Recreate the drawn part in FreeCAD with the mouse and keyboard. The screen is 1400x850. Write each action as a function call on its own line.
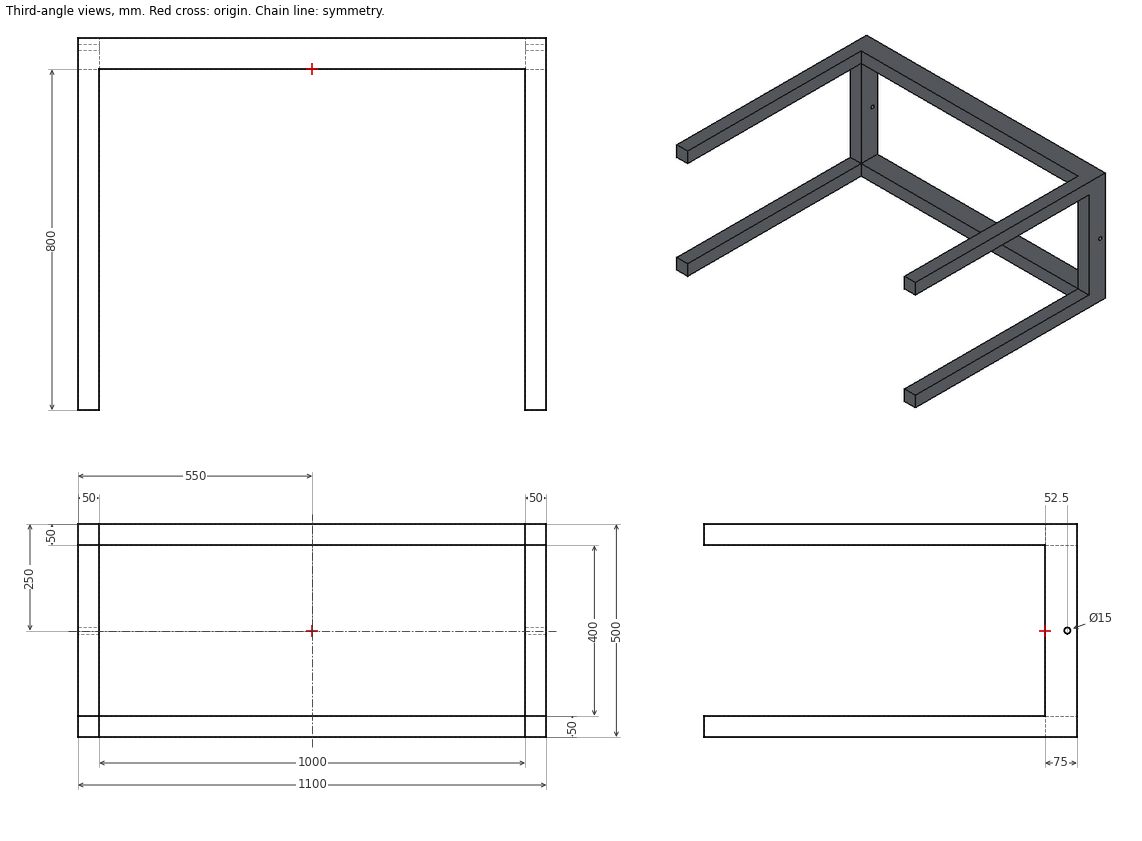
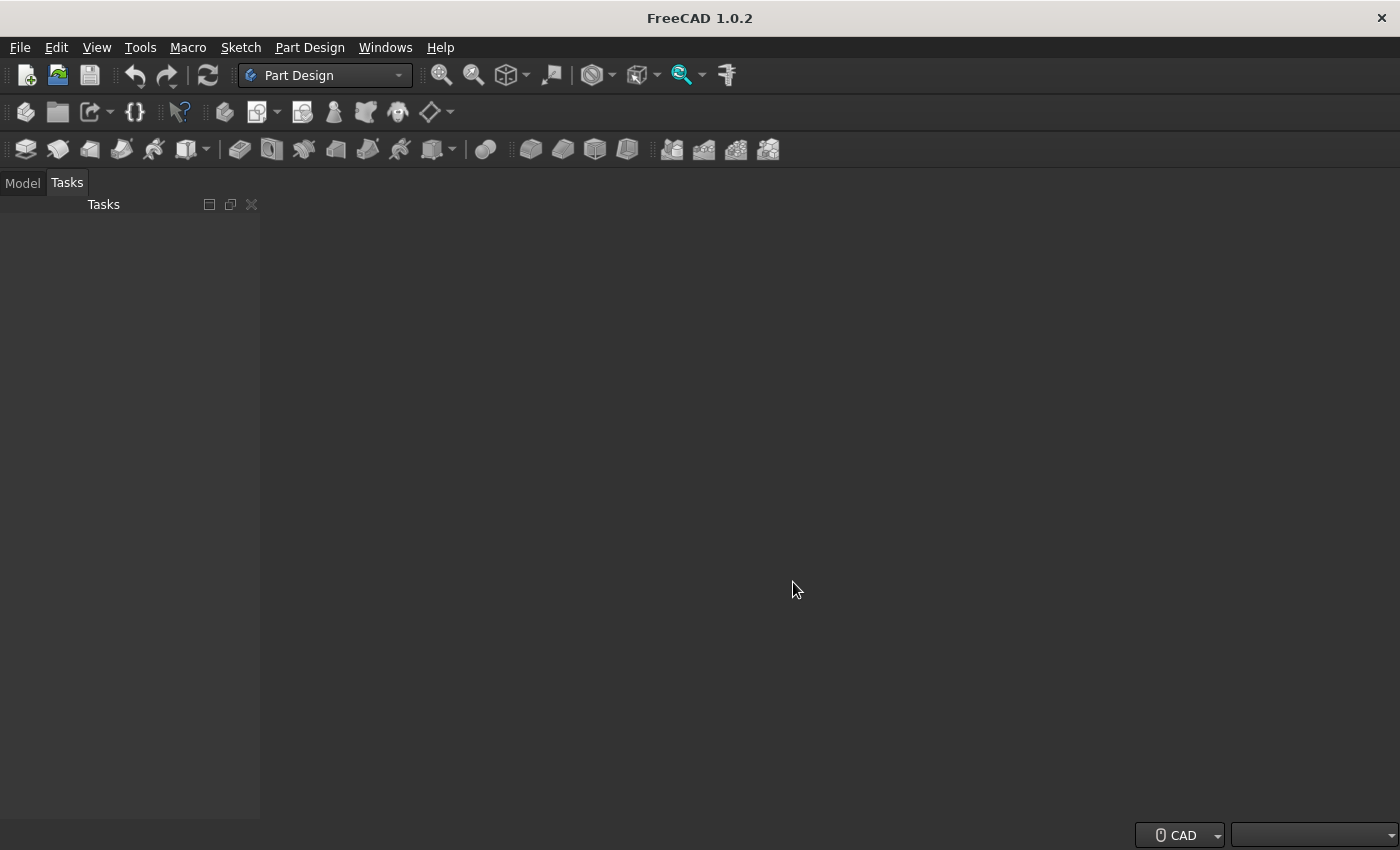
click(26, 76)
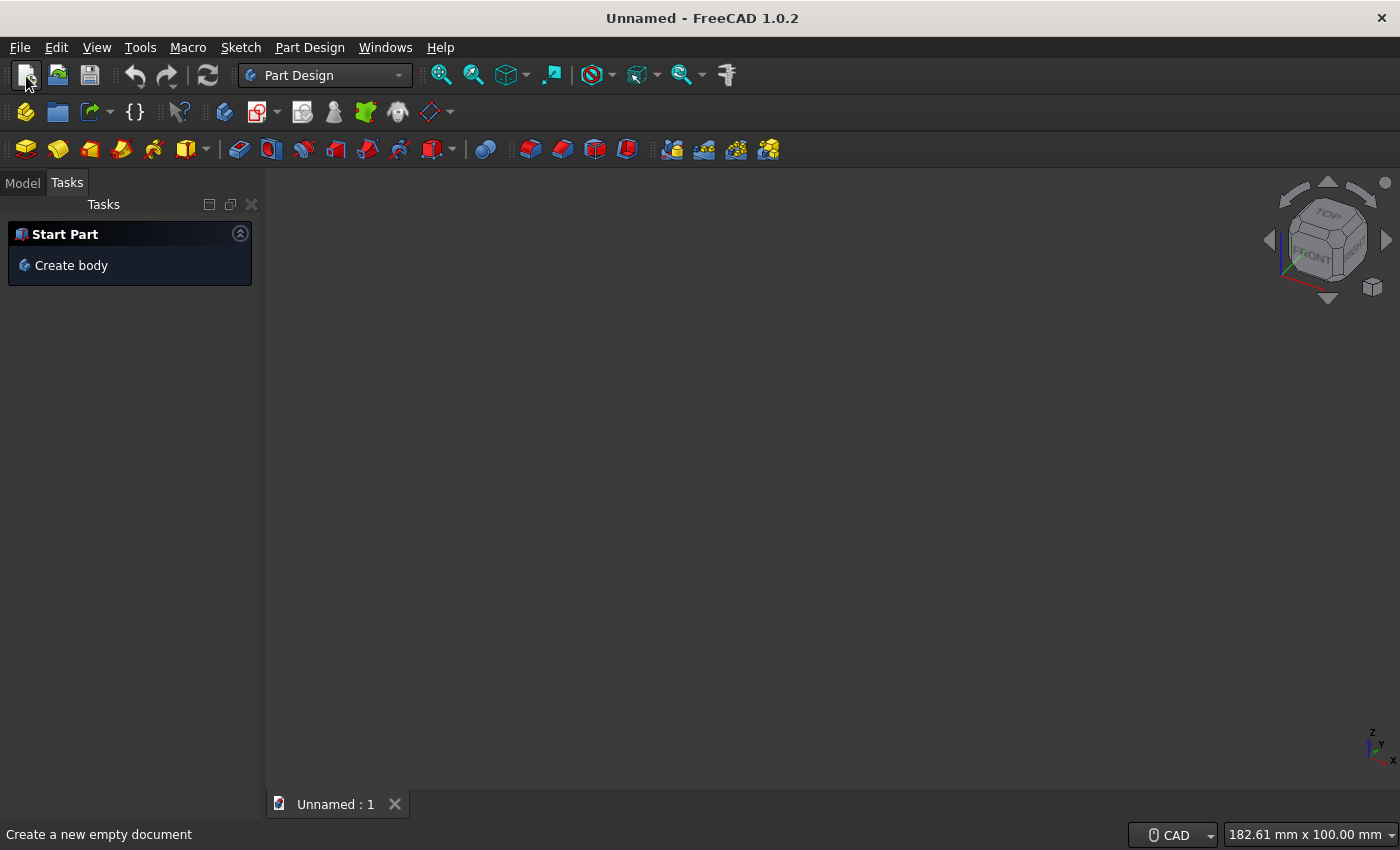
click(258, 112)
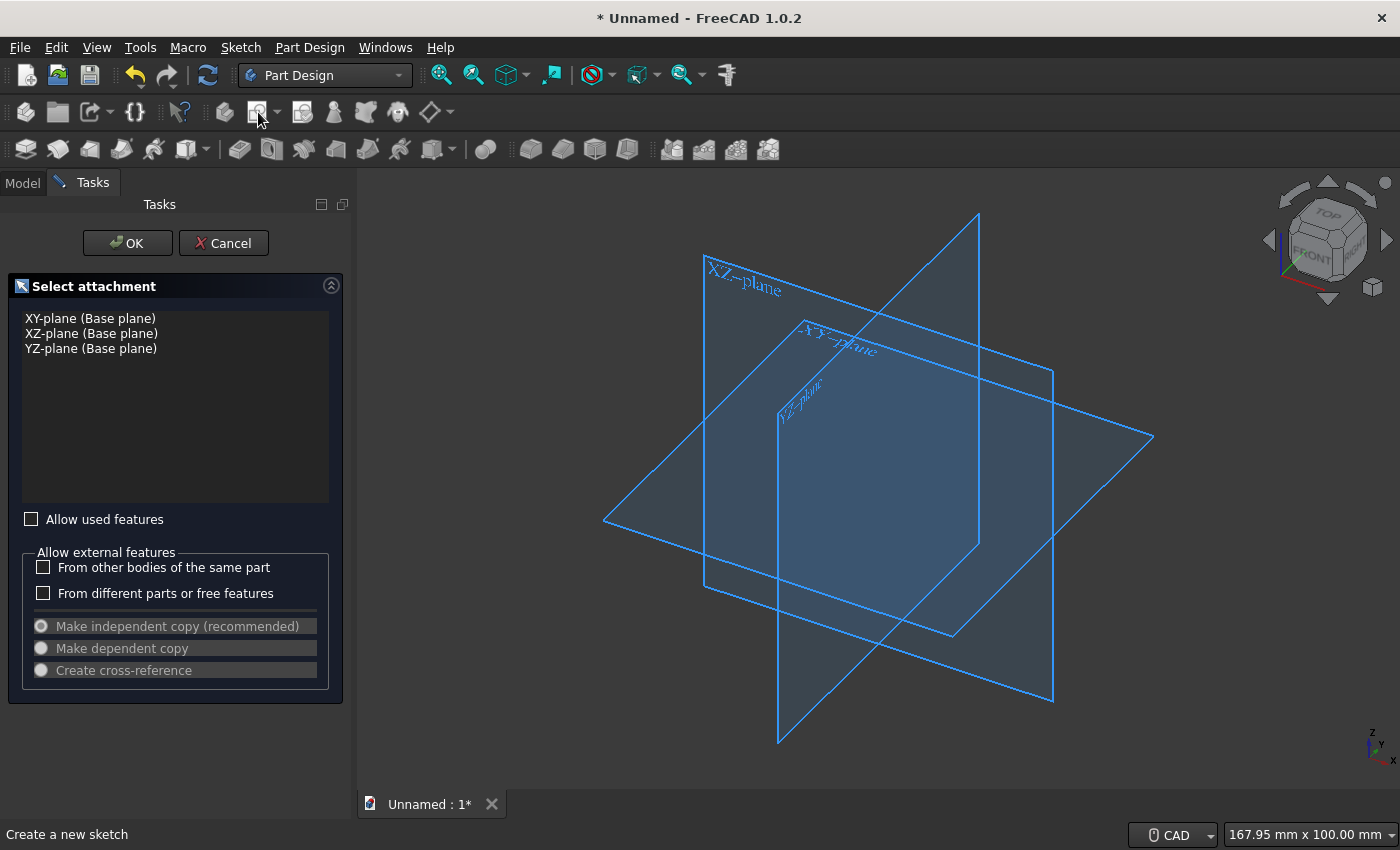
click(82, 334)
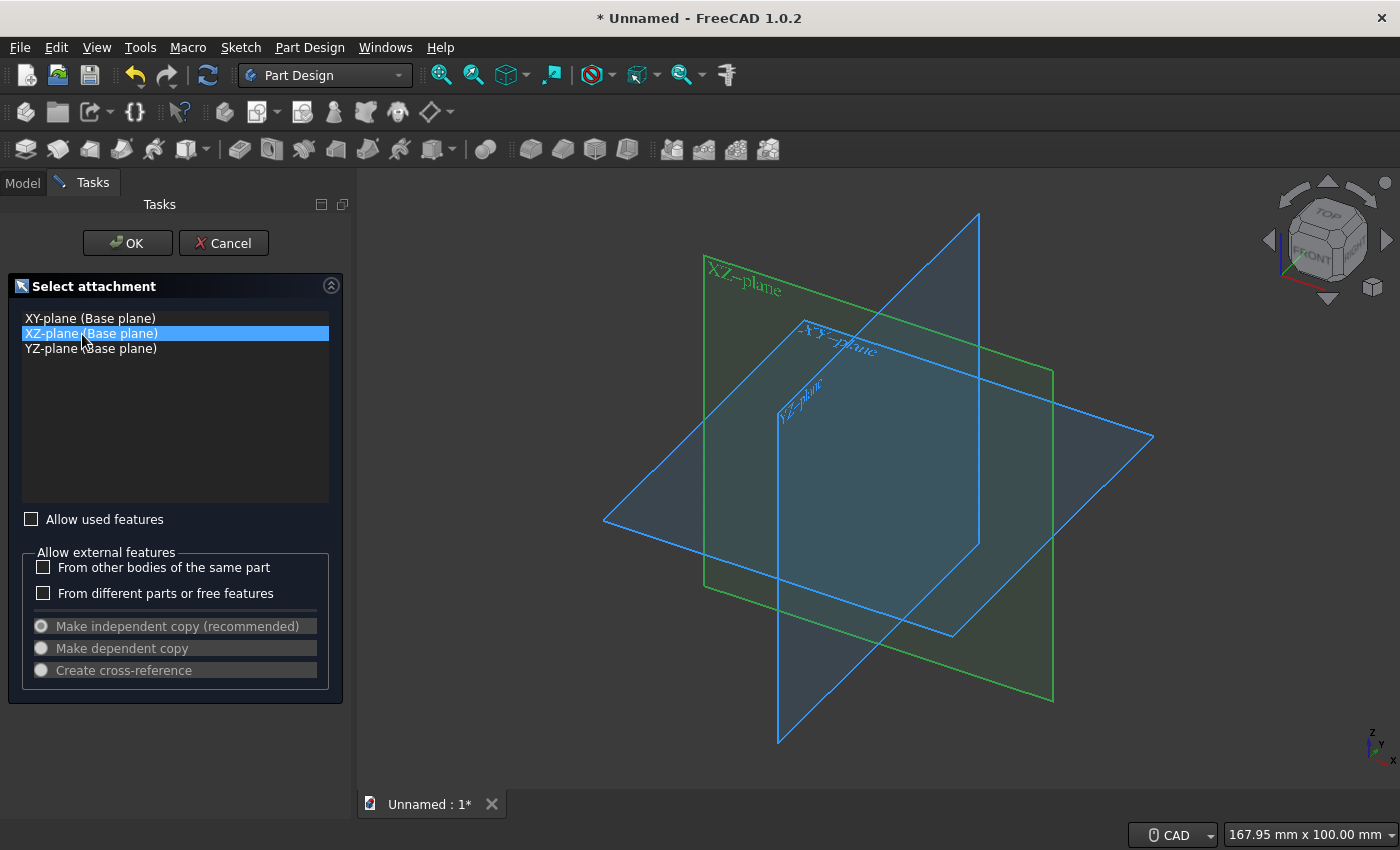
click(128, 243)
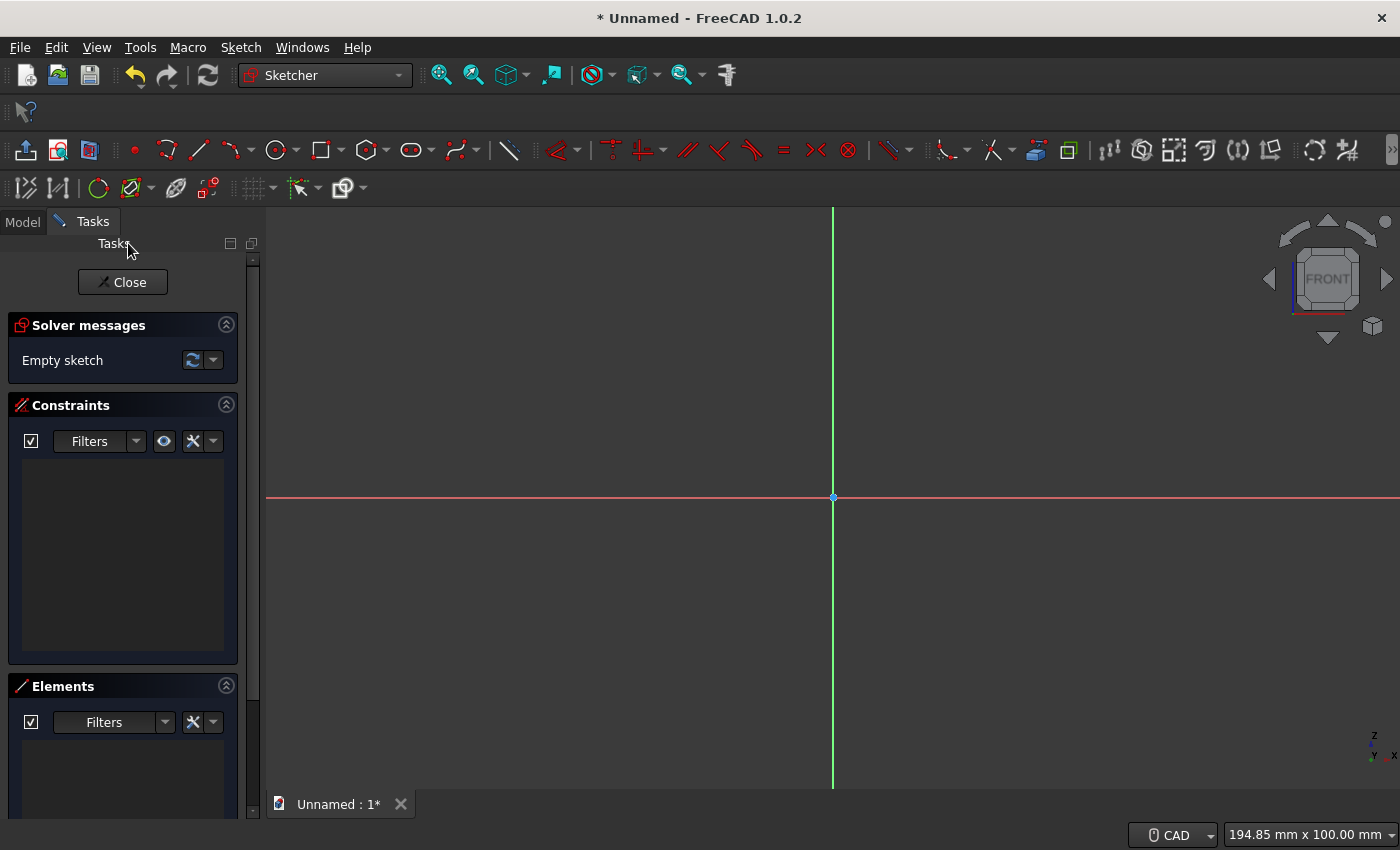
scroll(756, 498, down, 11)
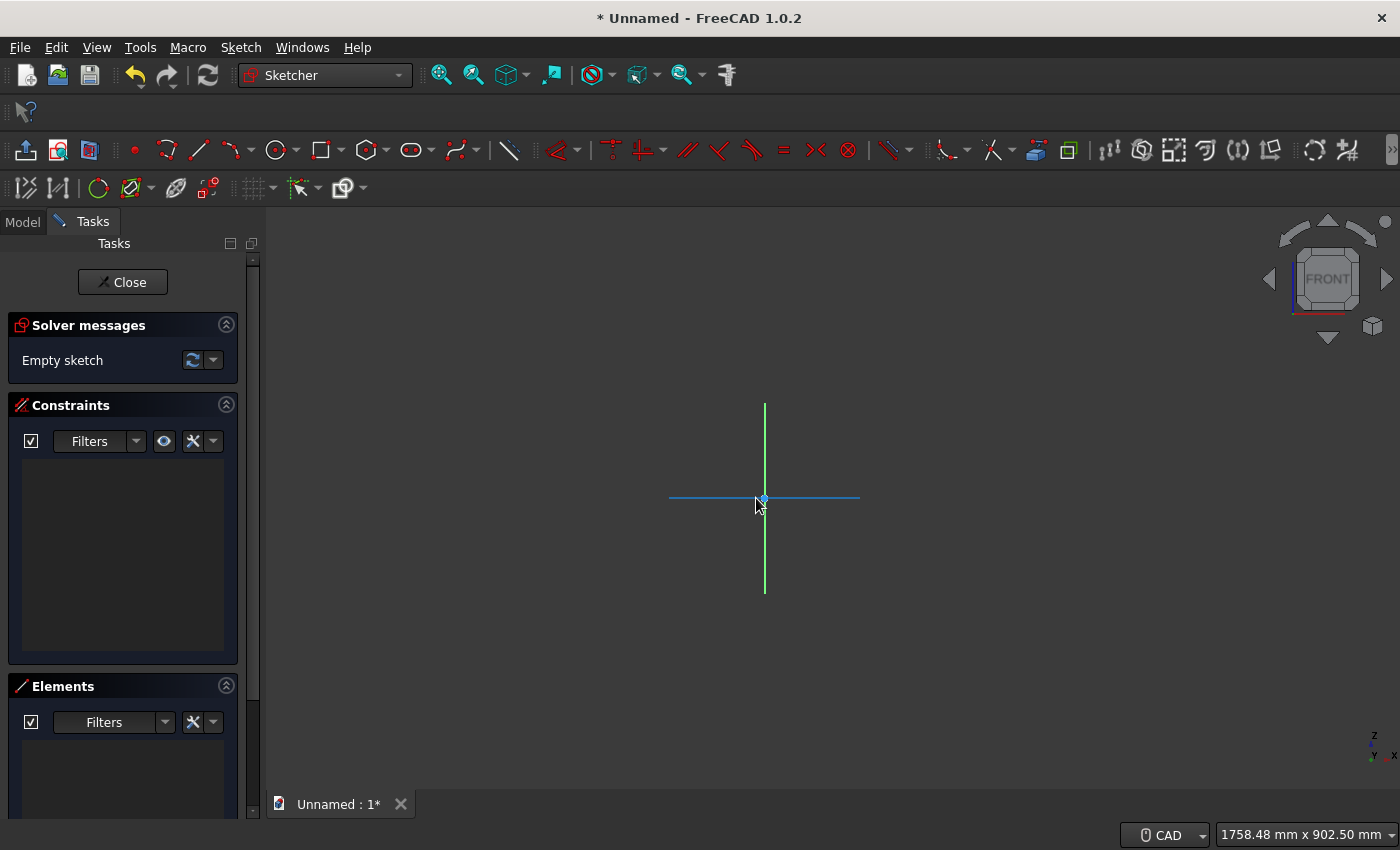
click(344, 150)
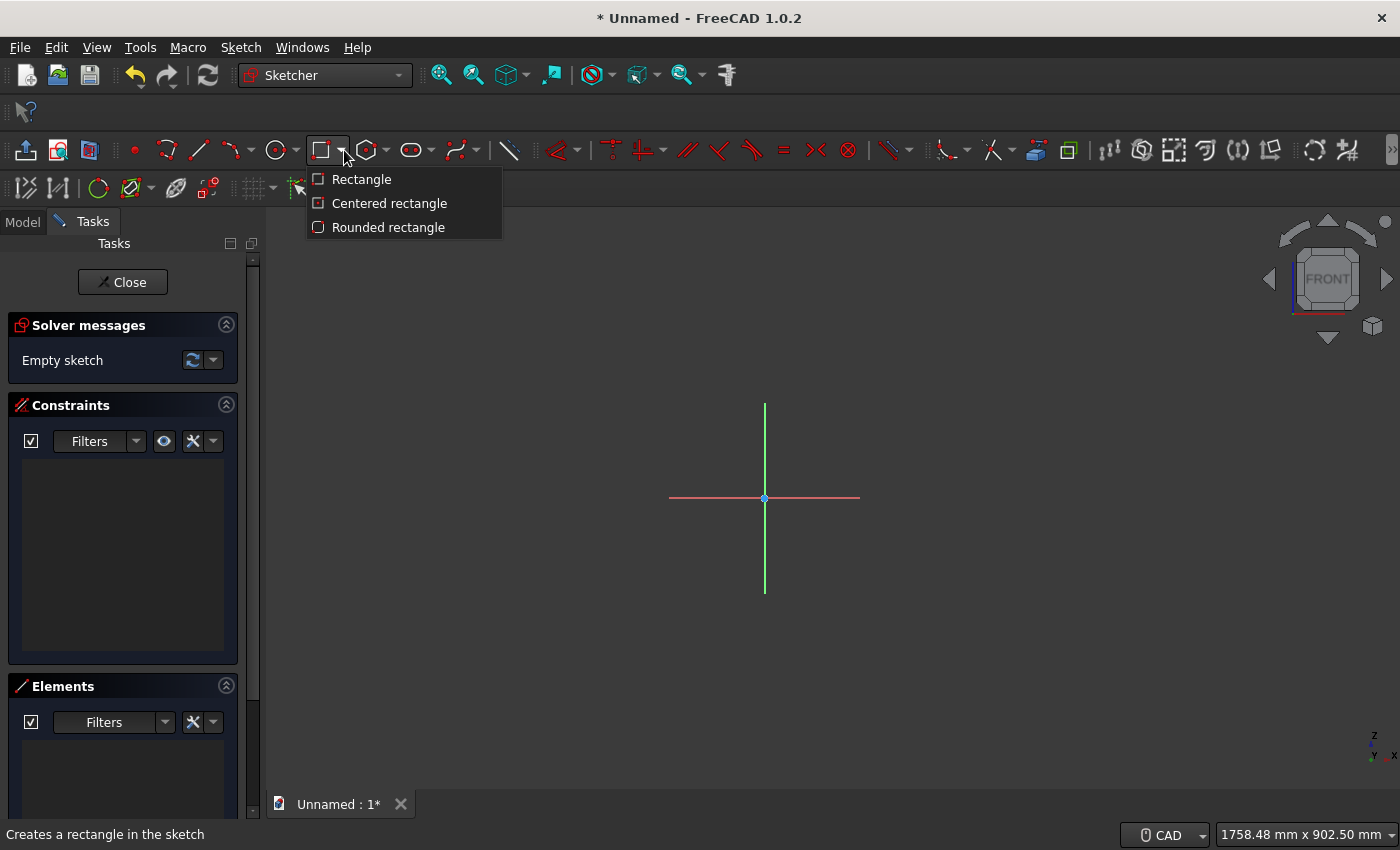
click(404, 203)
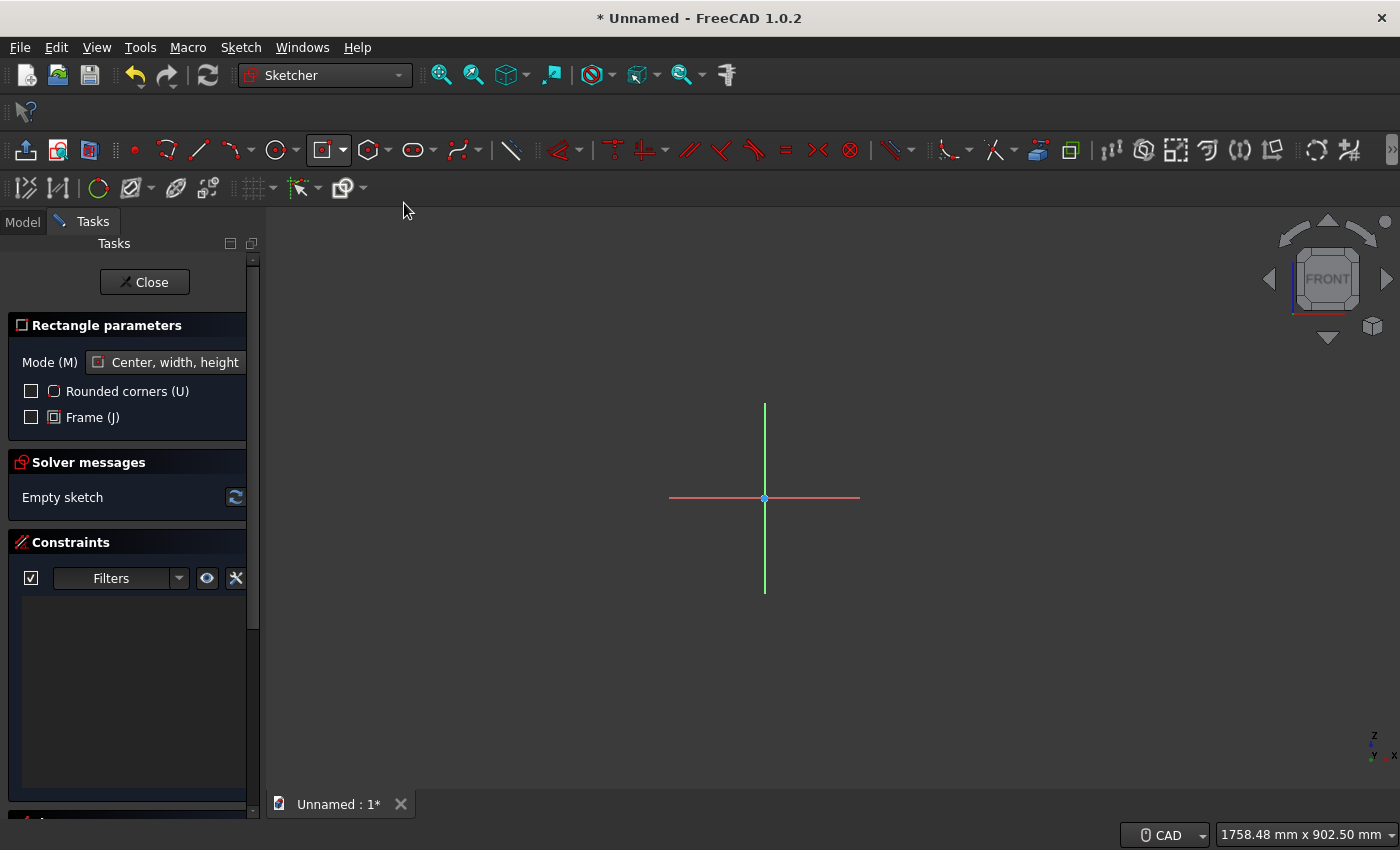
click(765, 498)
move(1120, 337)